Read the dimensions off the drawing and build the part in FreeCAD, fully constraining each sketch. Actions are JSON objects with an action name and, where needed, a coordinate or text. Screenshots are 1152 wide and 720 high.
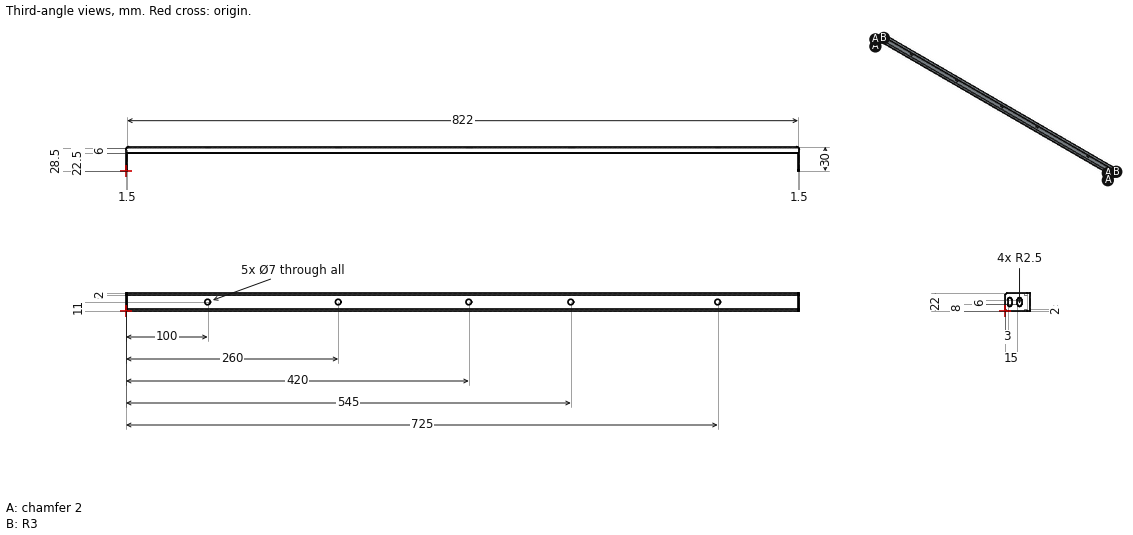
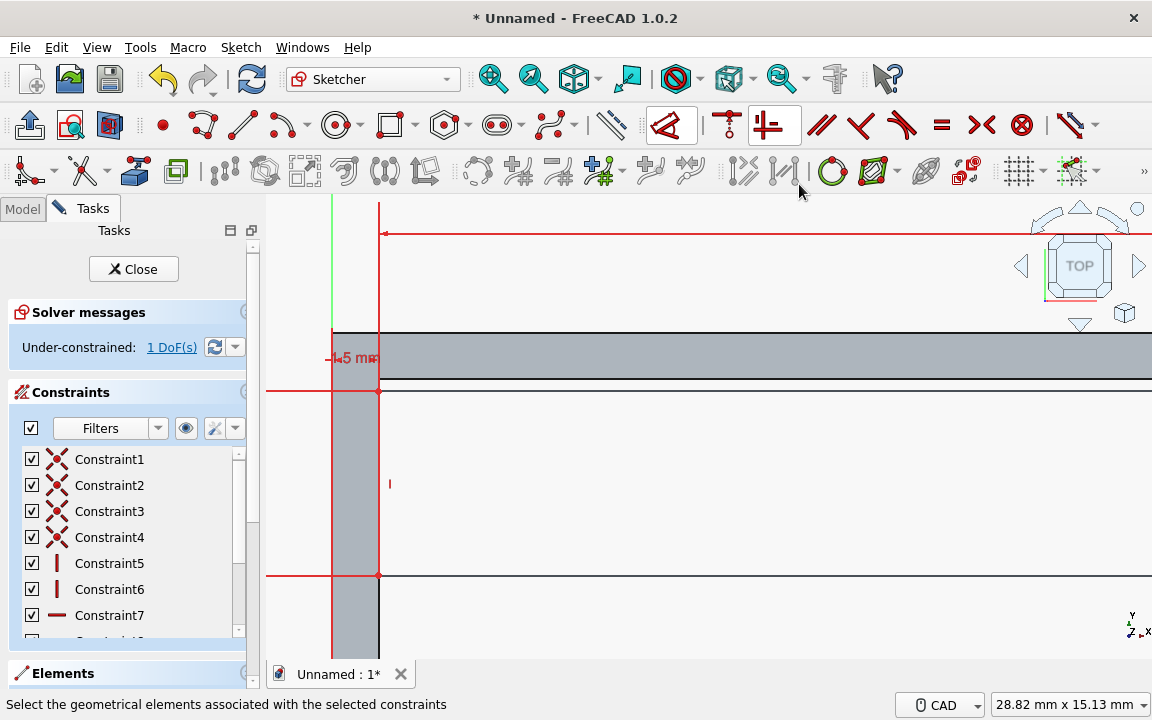
{"action": "scroll", "coordinate": [640, 426], "scroll_direction": "down", "scroll_amount": 15}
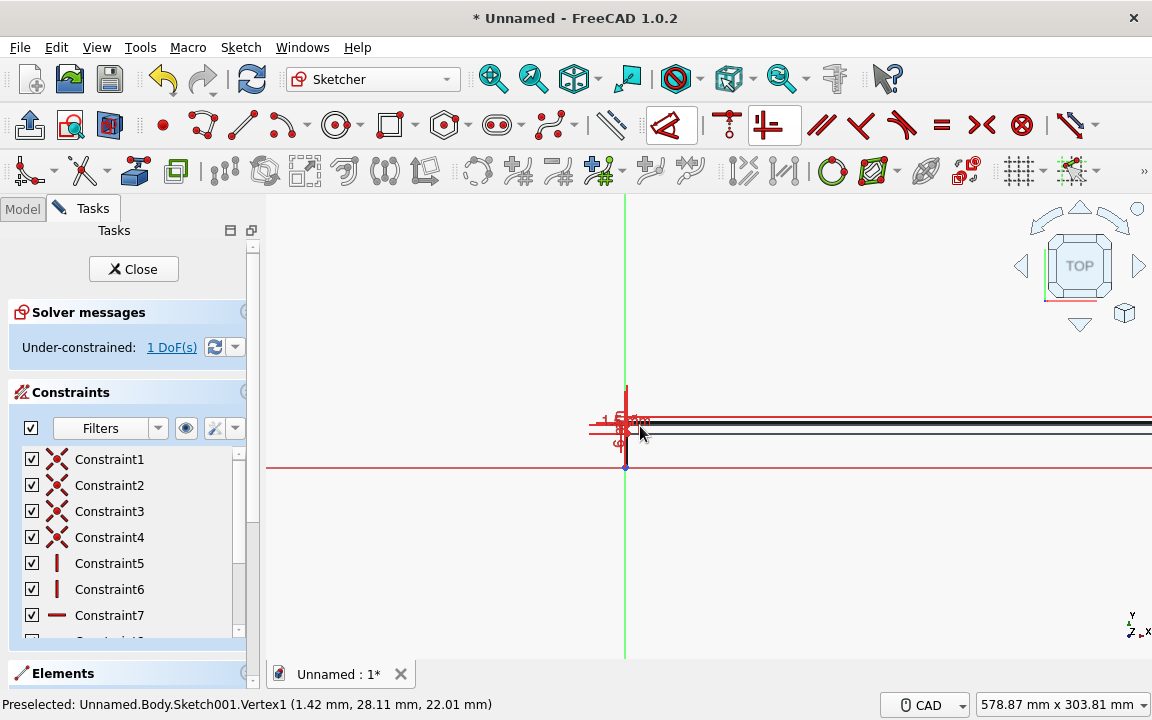
{"action": "scroll", "coordinate": [294, 415], "scroll_direction": "down", "scroll_amount": 5}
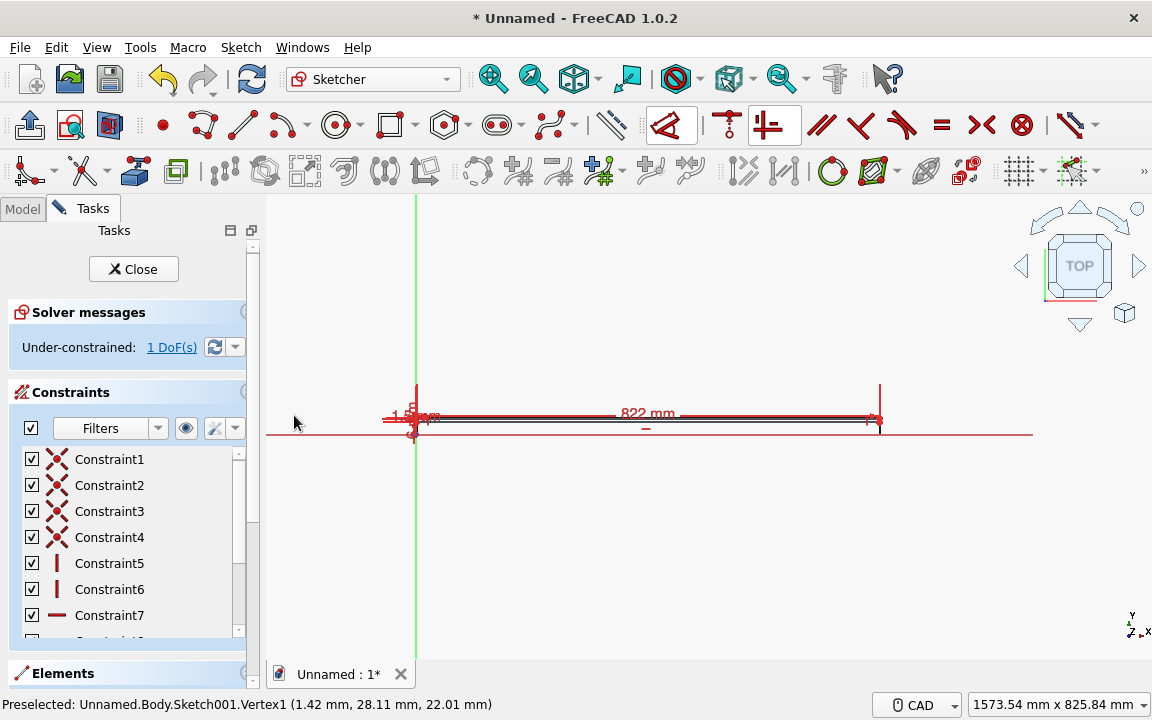
{"action": "scroll", "coordinate": [417, 419], "scroll_direction": "up", "scroll_amount": 7}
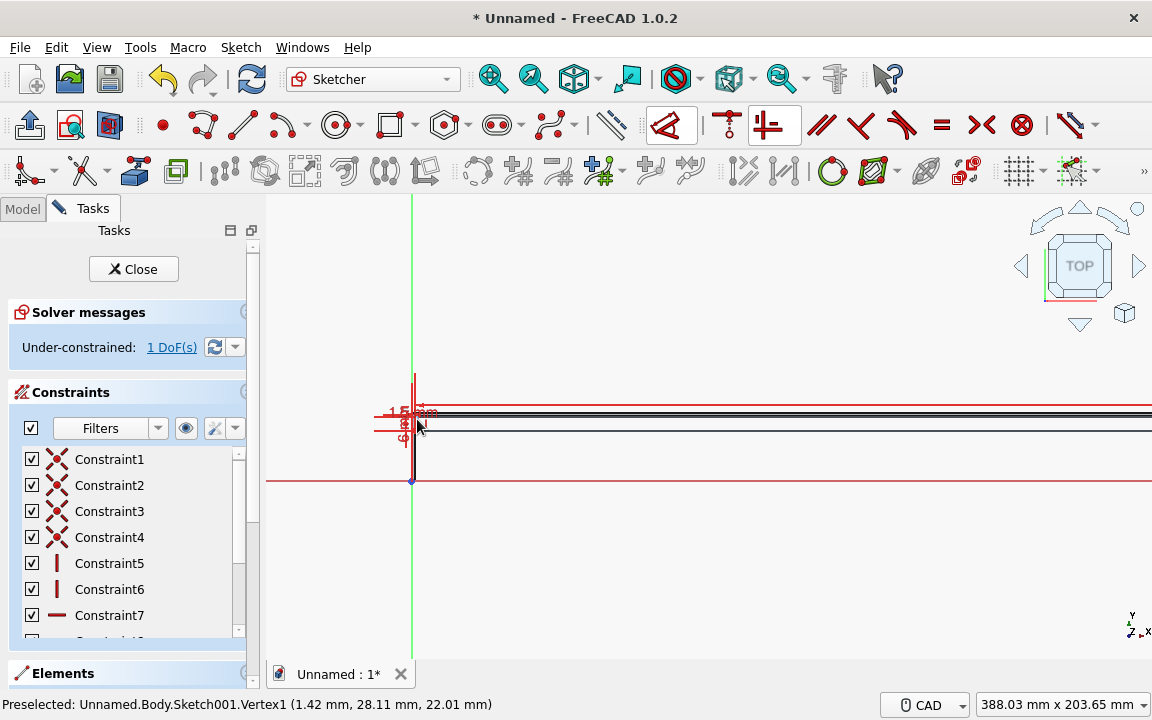
{"action": "left_click", "coordinate": [415, 417]}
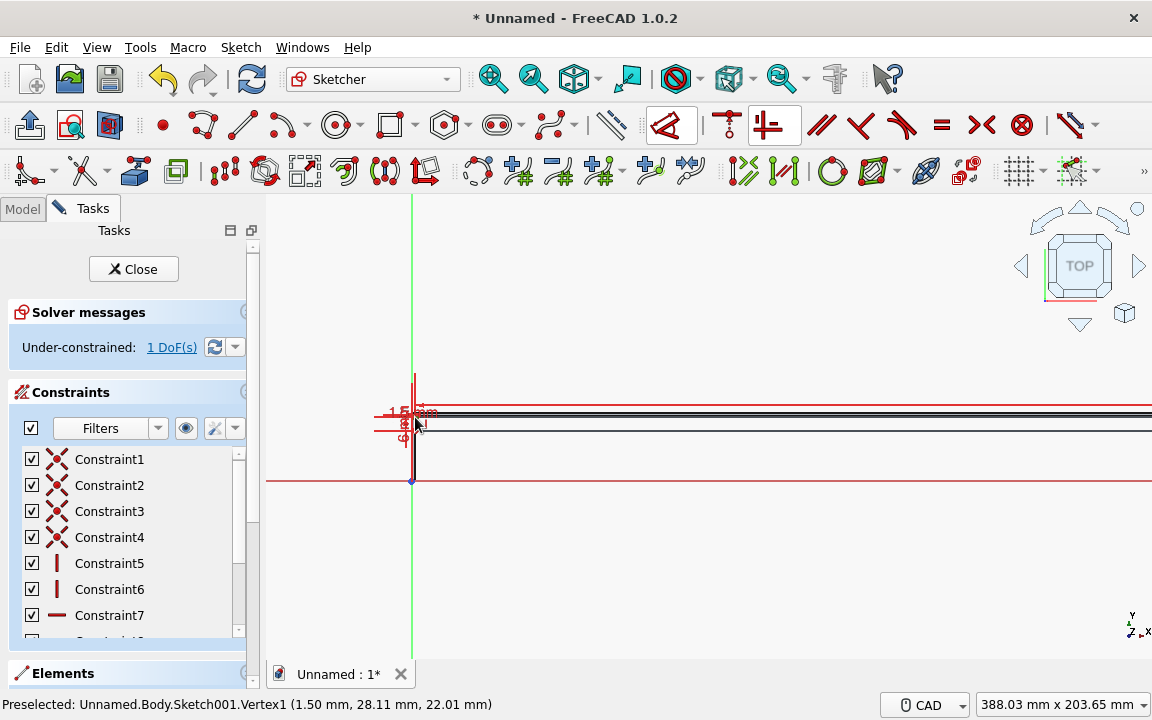
{"action": "left_click", "coordinate": [692, 126]}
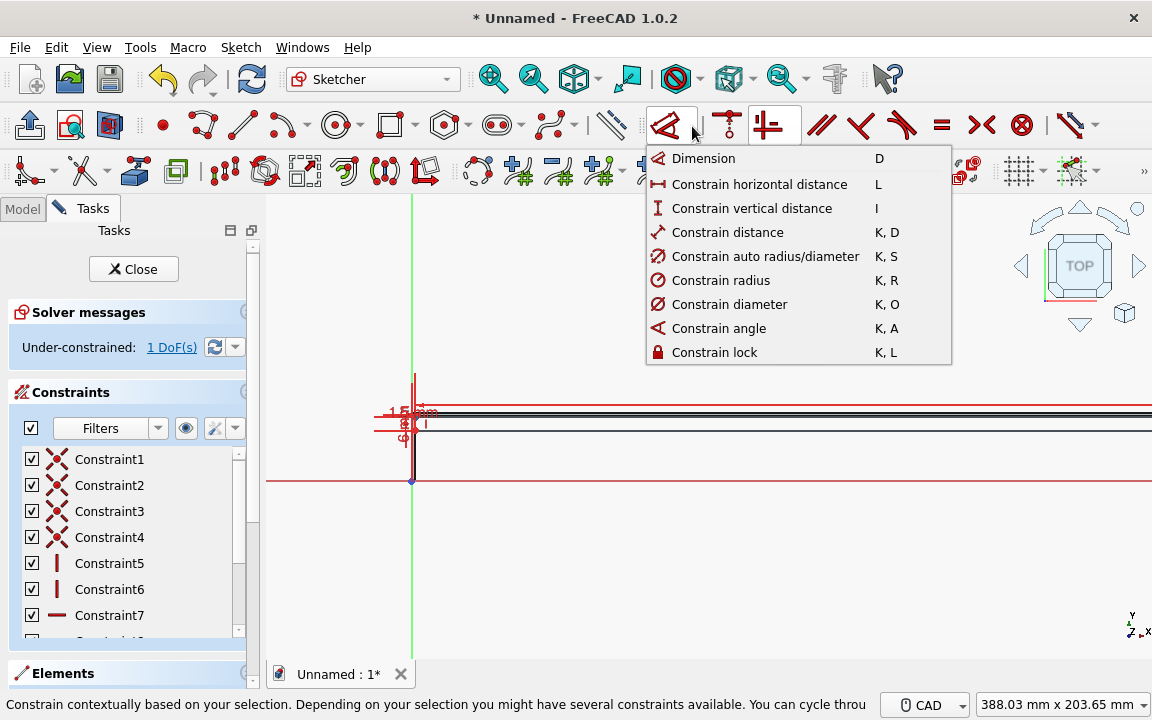
{"action": "left_click", "coordinate": [799, 208]}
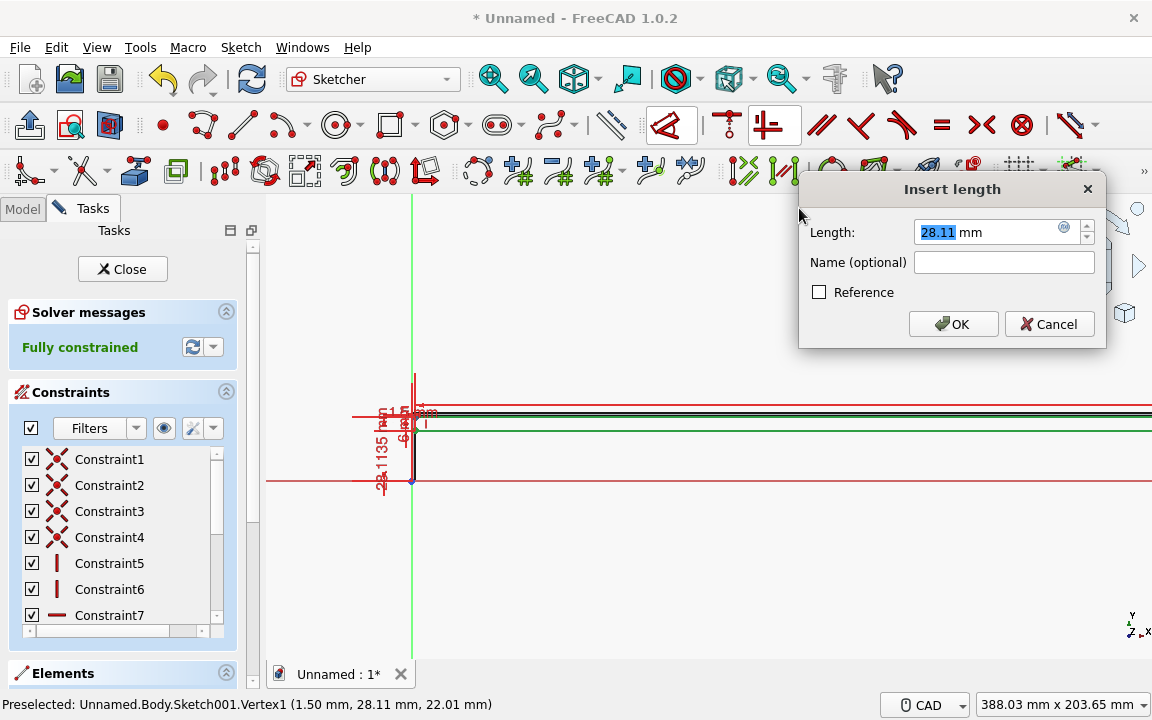
{"action": "type", "text": "28.5"}
{"action": "key", "text": "Return"}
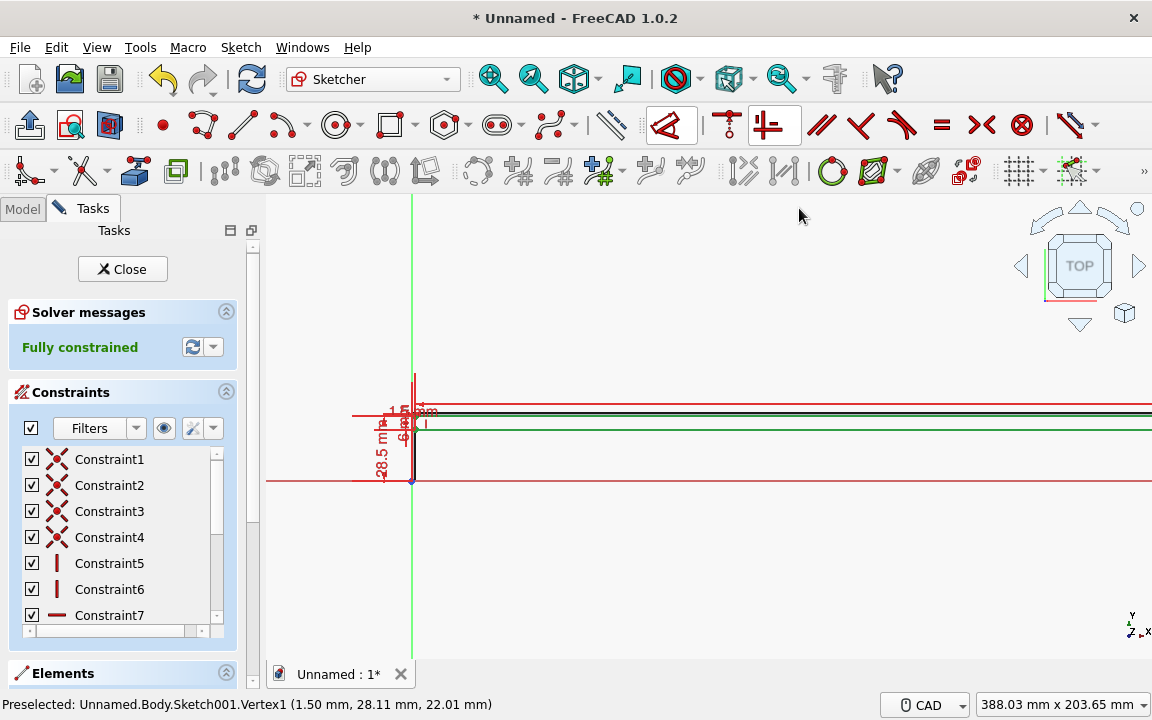
{"action": "left_click", "coordinate": [123, 269]}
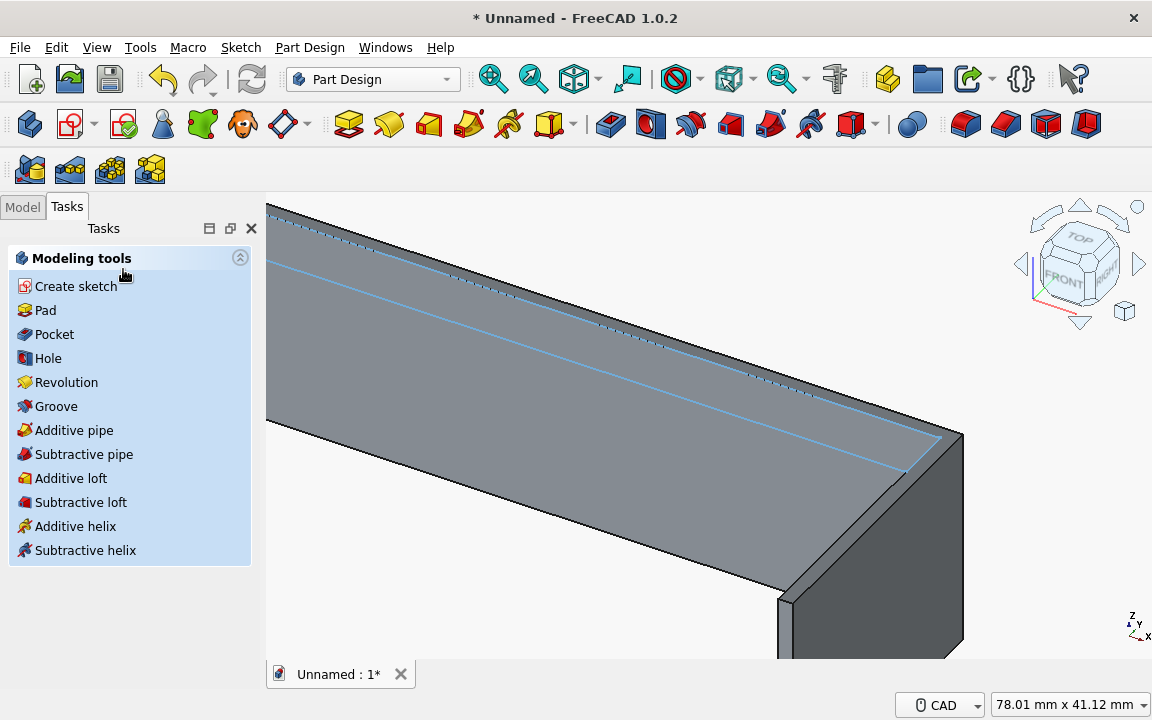
{"action": "left_click", "coordinate": [350, 124]}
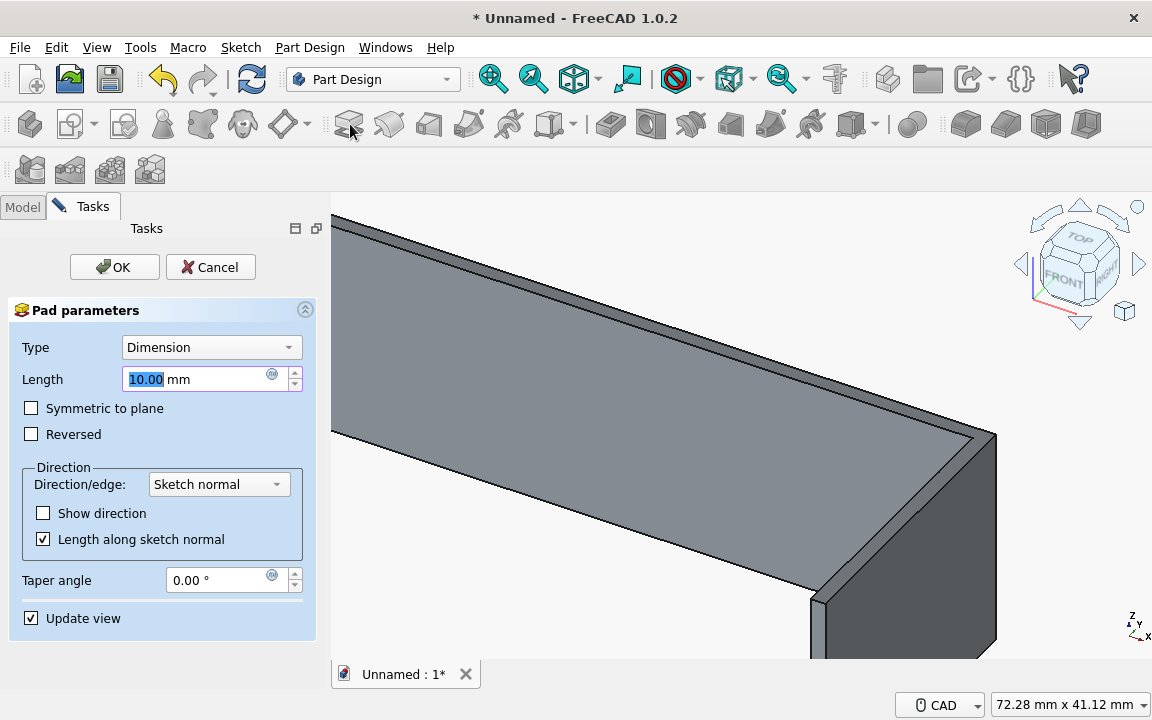
{"action": "type", "text": "2"}
{"action": "key", "text": "Tab"}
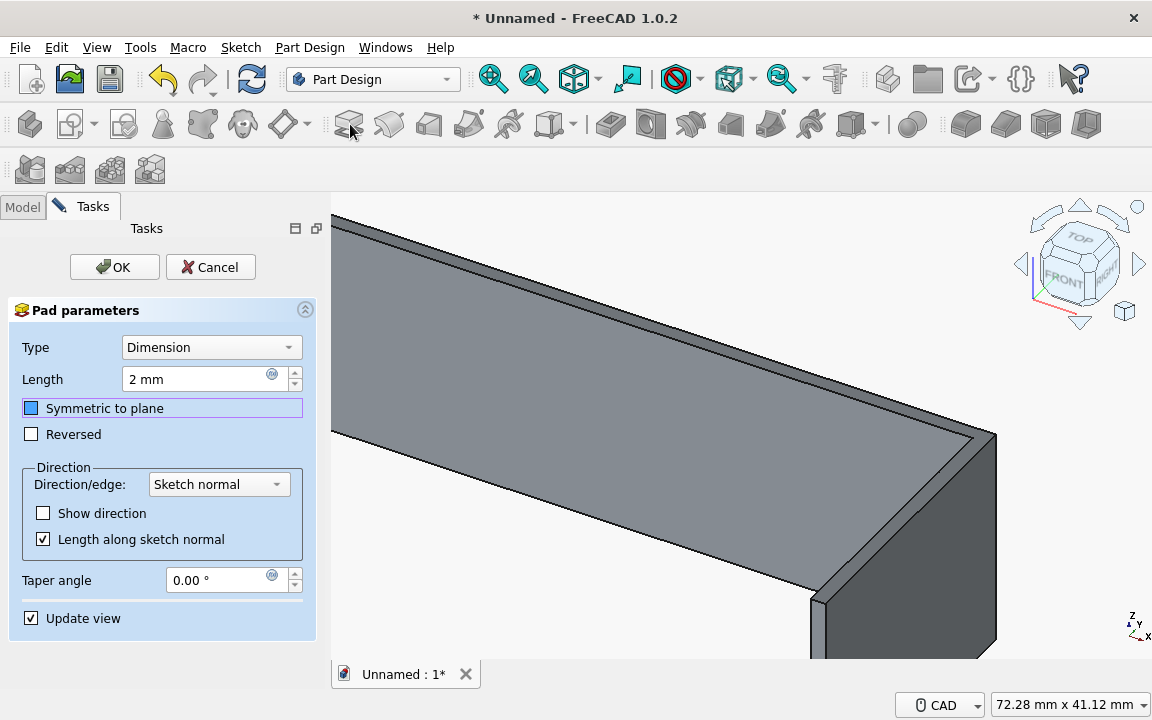
{"action": "left_click", "coordinate": [30, 434]}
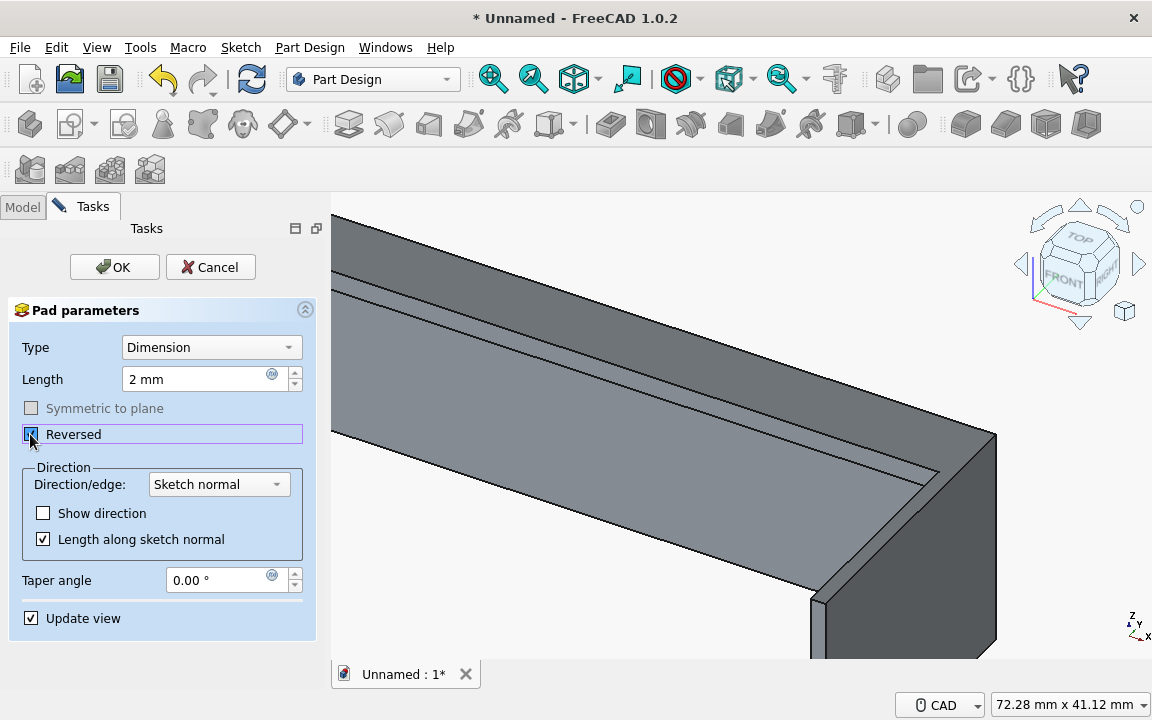
{"action": "left_click", "coordinate": [115, 267]}